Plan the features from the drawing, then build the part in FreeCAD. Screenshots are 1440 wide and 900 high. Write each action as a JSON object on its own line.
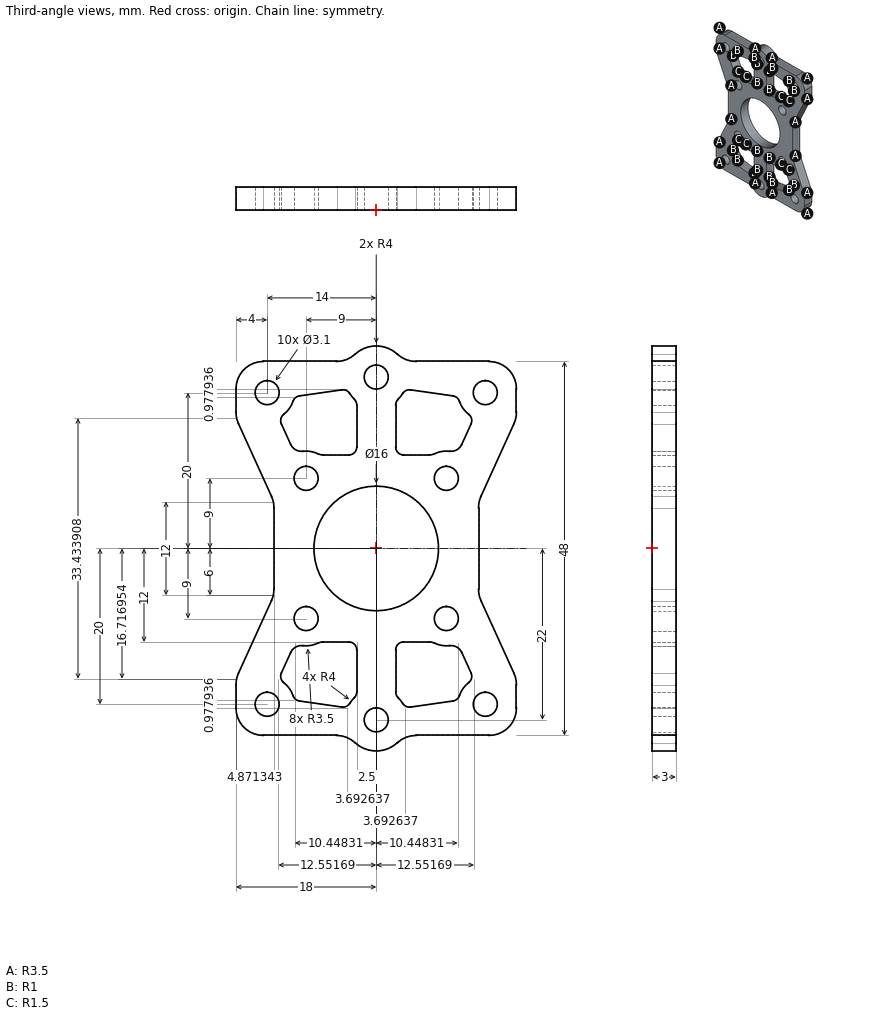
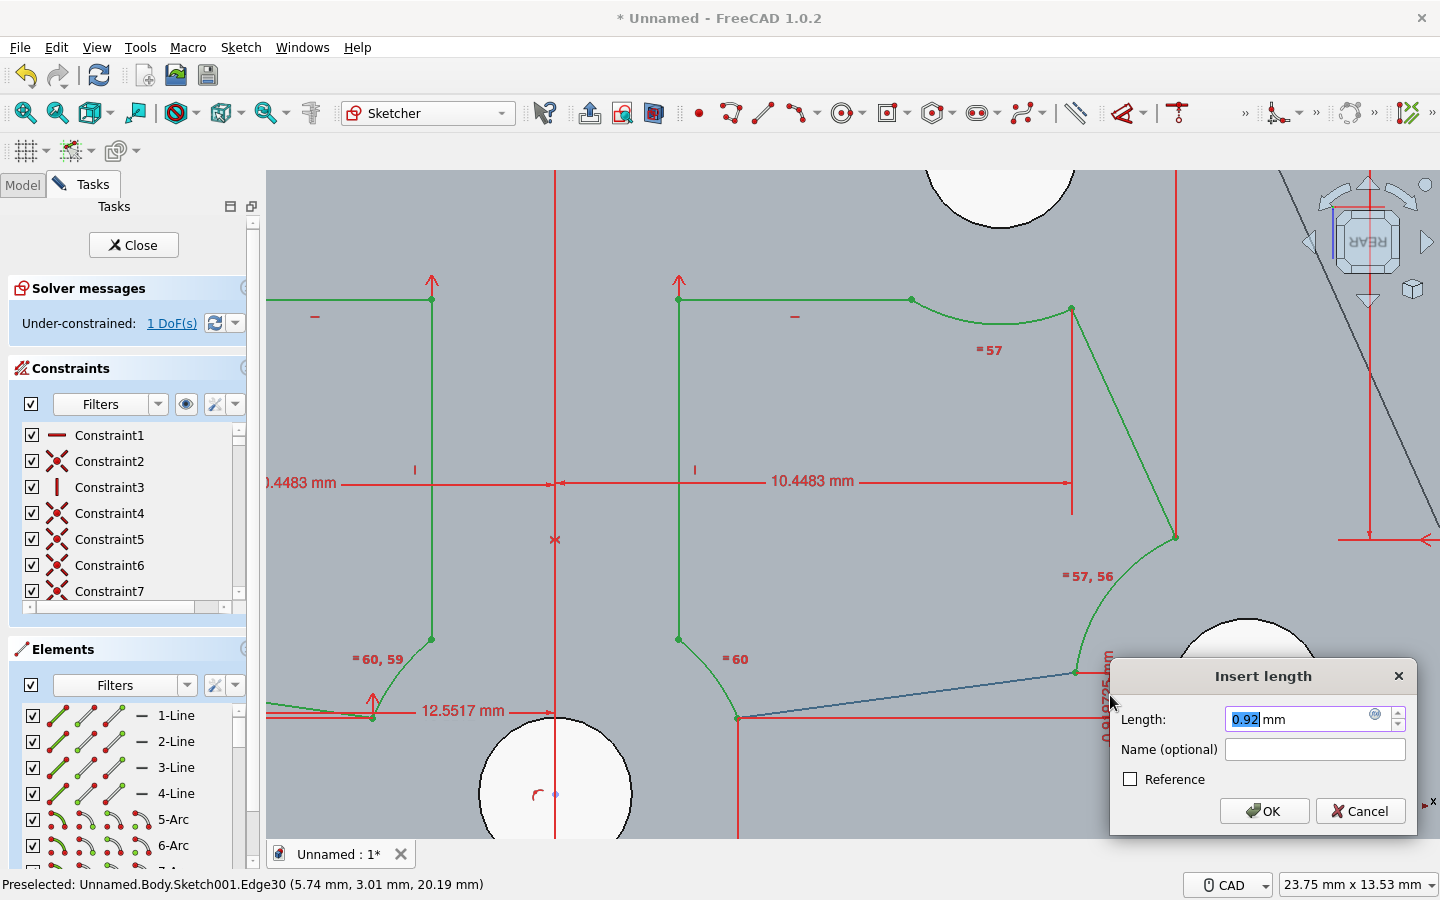
{"action": "type", "text": "0.977936"}
{"action": "key", "text": "Return"}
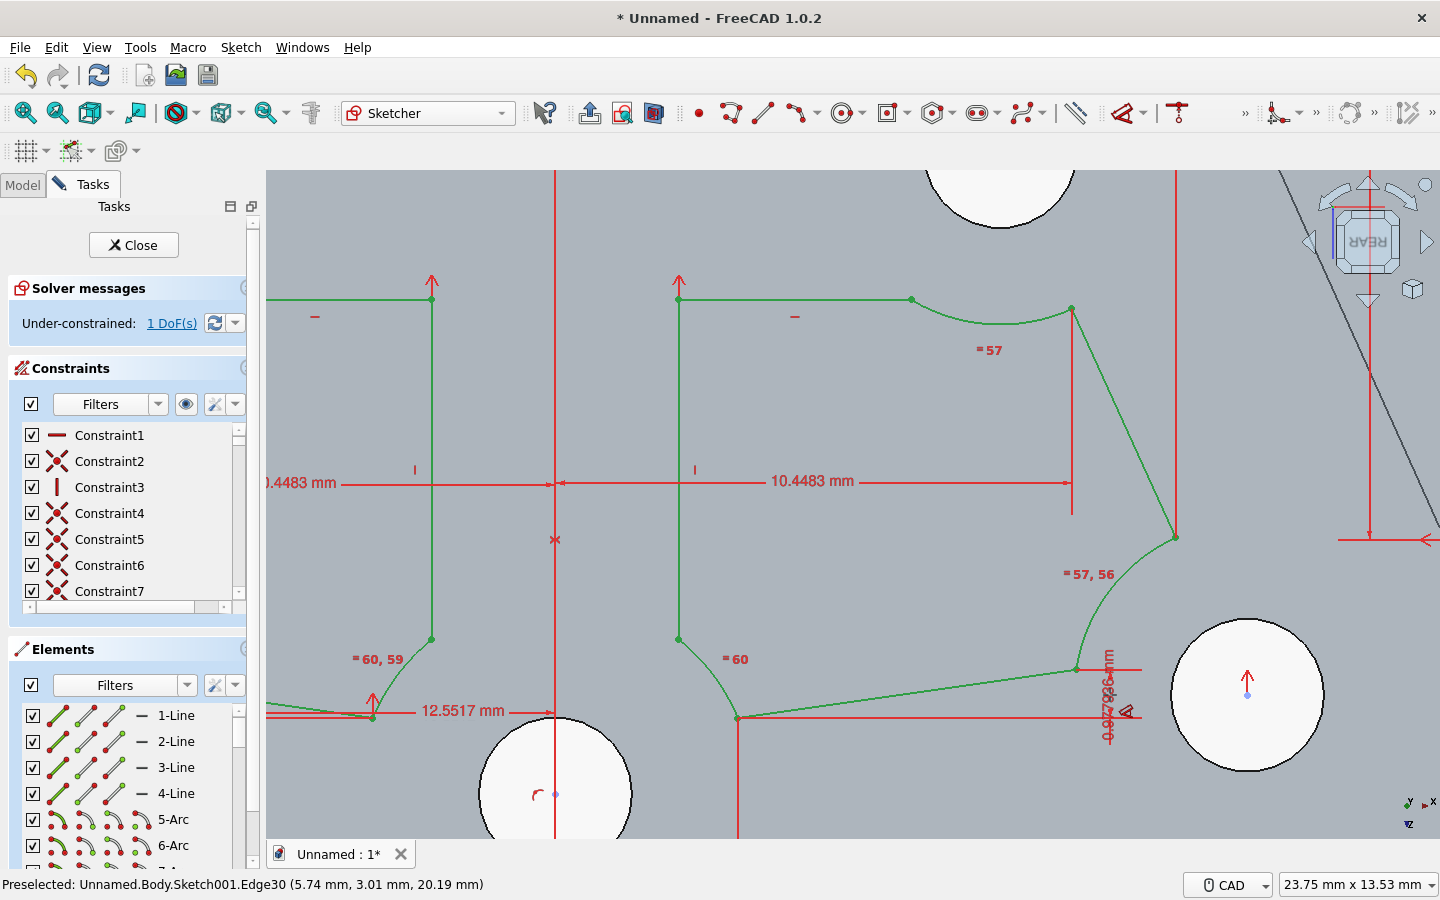
{"action": "scroll", "coordinate": [842, 706], "scroll_direction": "down", "scroll_amount": 8}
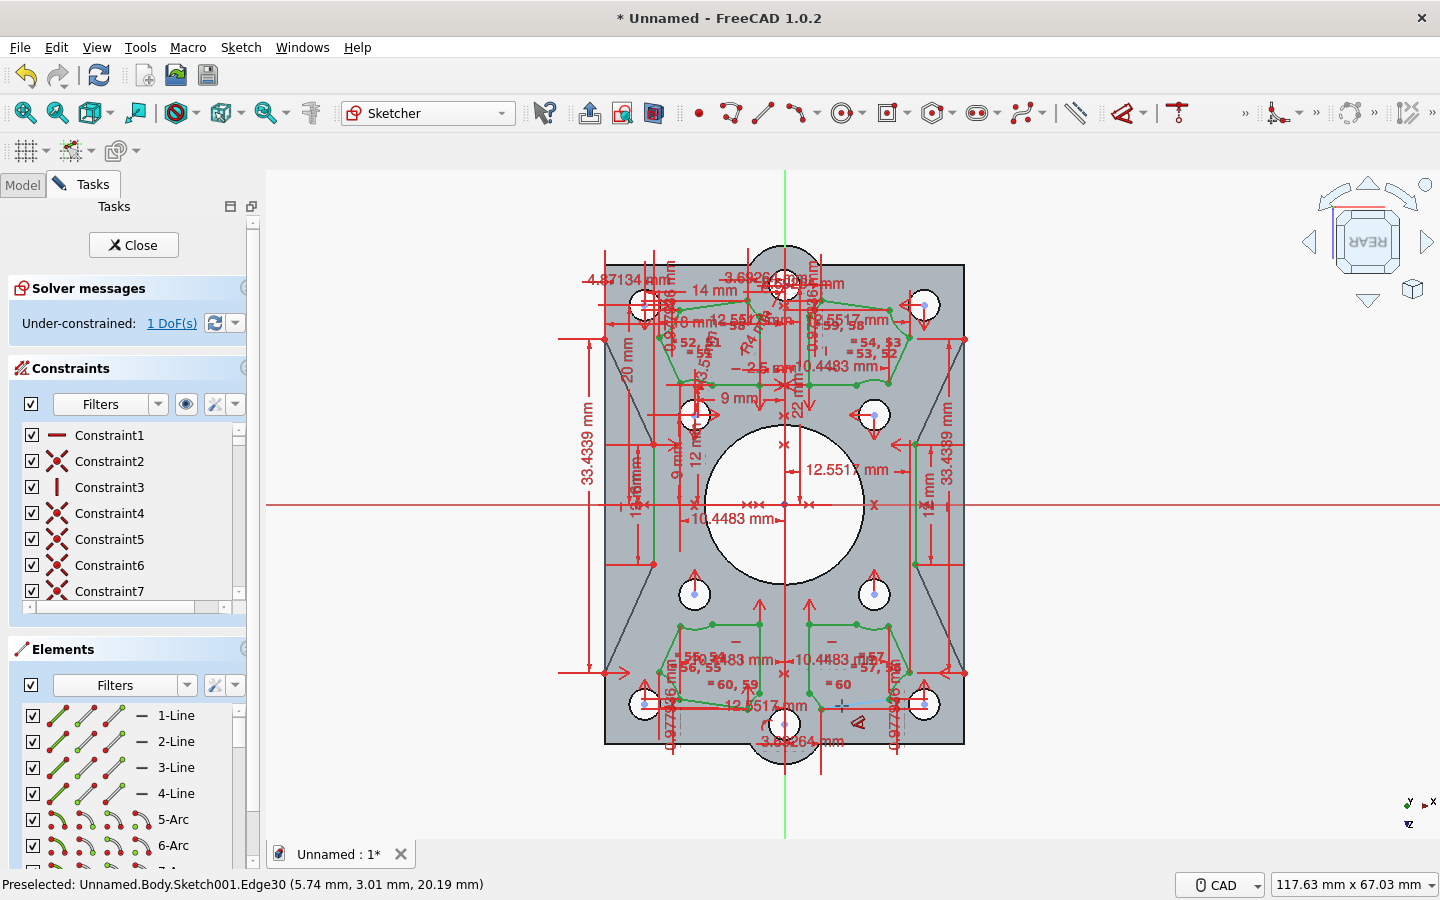
{"action": "left_click", "coordinate": [605, 339]}
{"action": "left_click", "coordinate": [571, 422]}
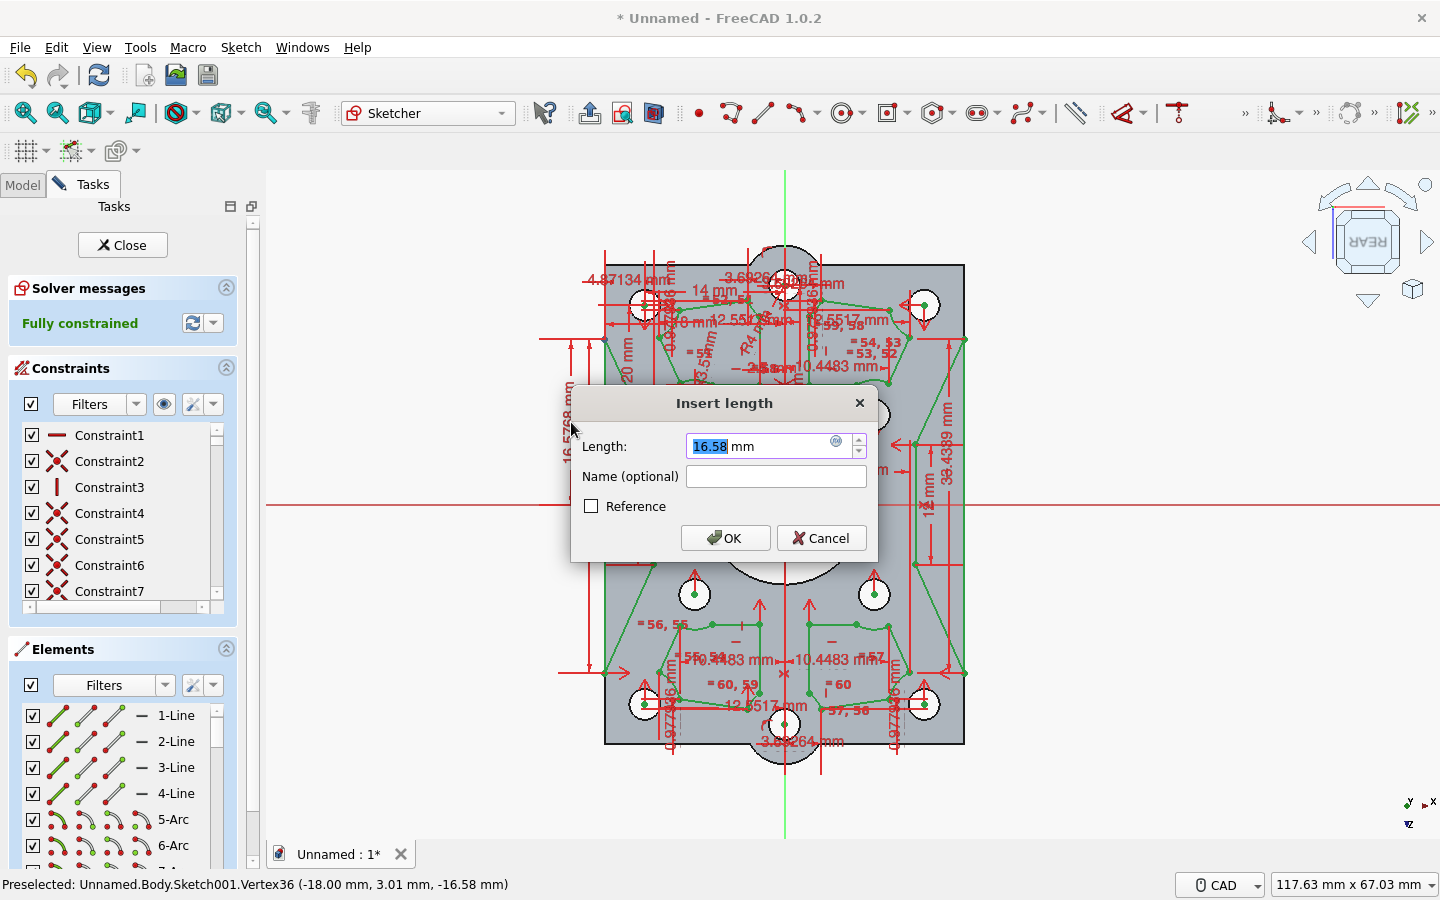
{"action": "type", "text": "16.716954"}
{"action": "key", "text": "Return"}
{"action": "key", "text": "Escape"}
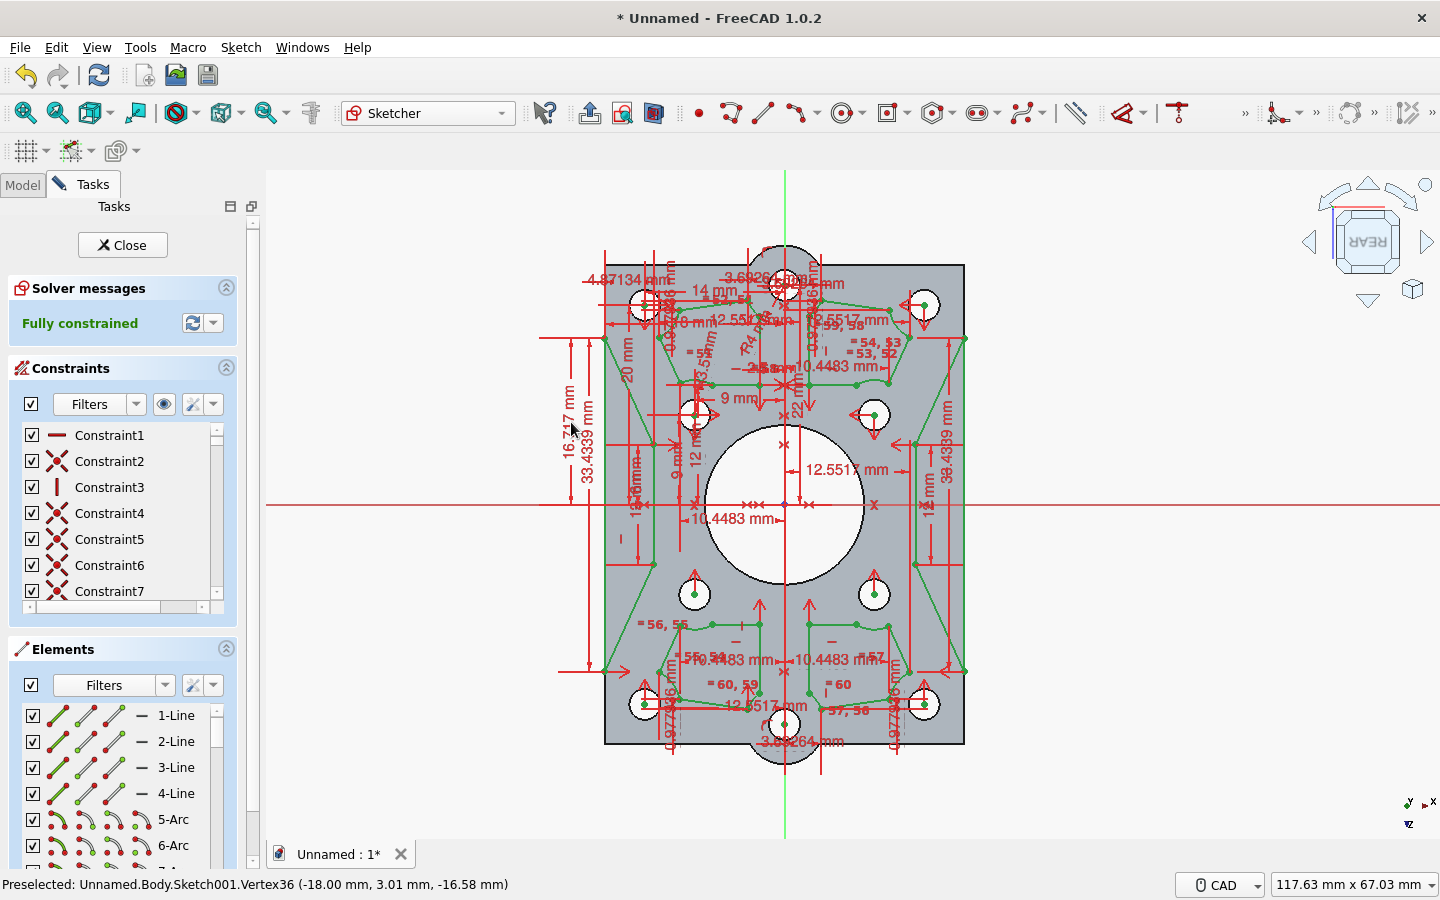
{"action": "left_click", "coordinate": [123, 245]}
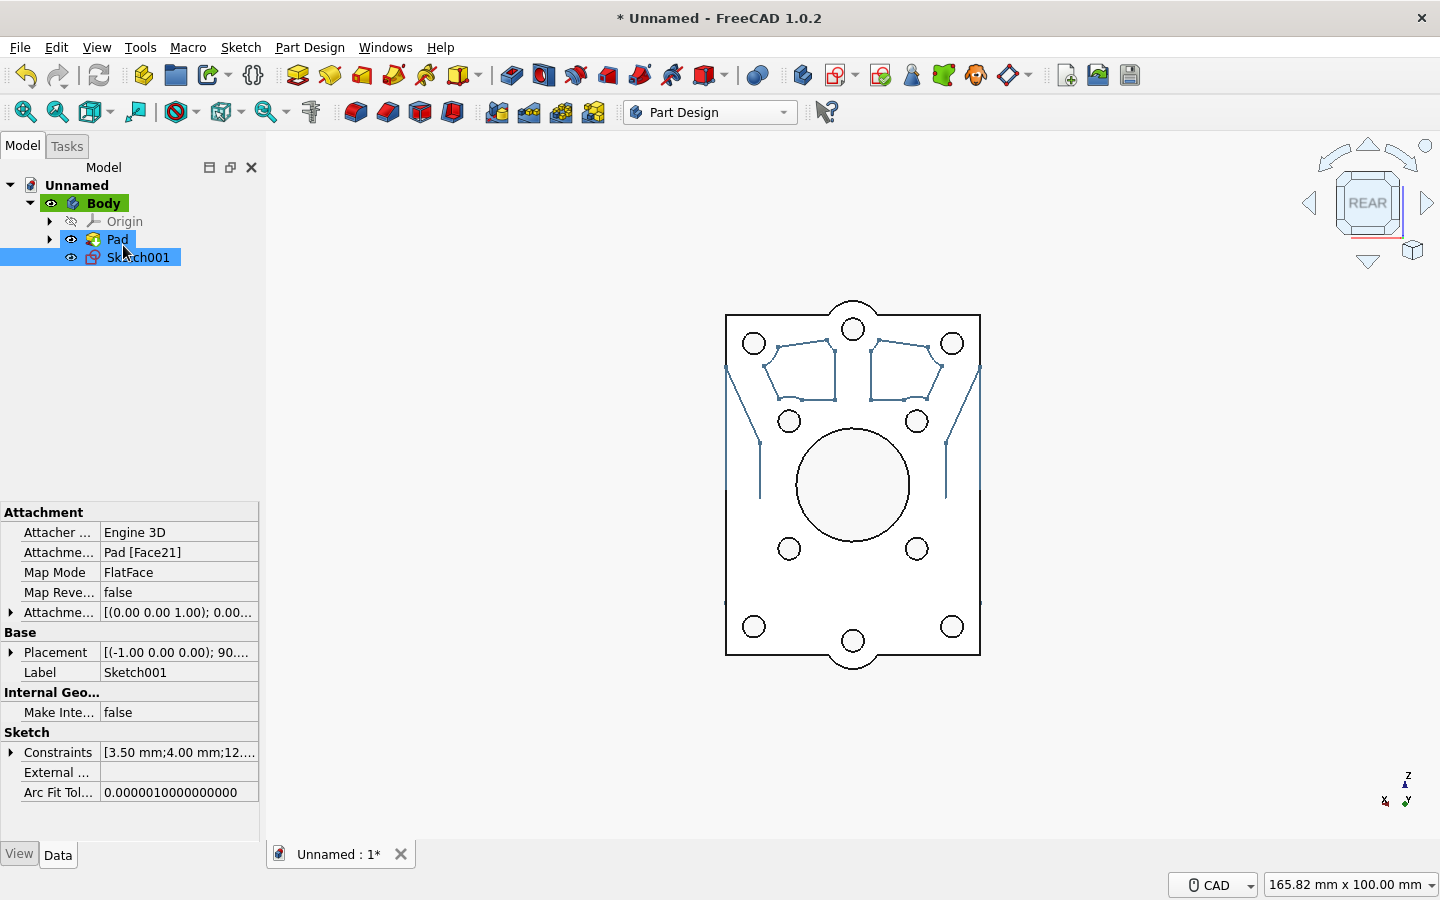
{"action": "left_click", "coordinate": [512, 76]}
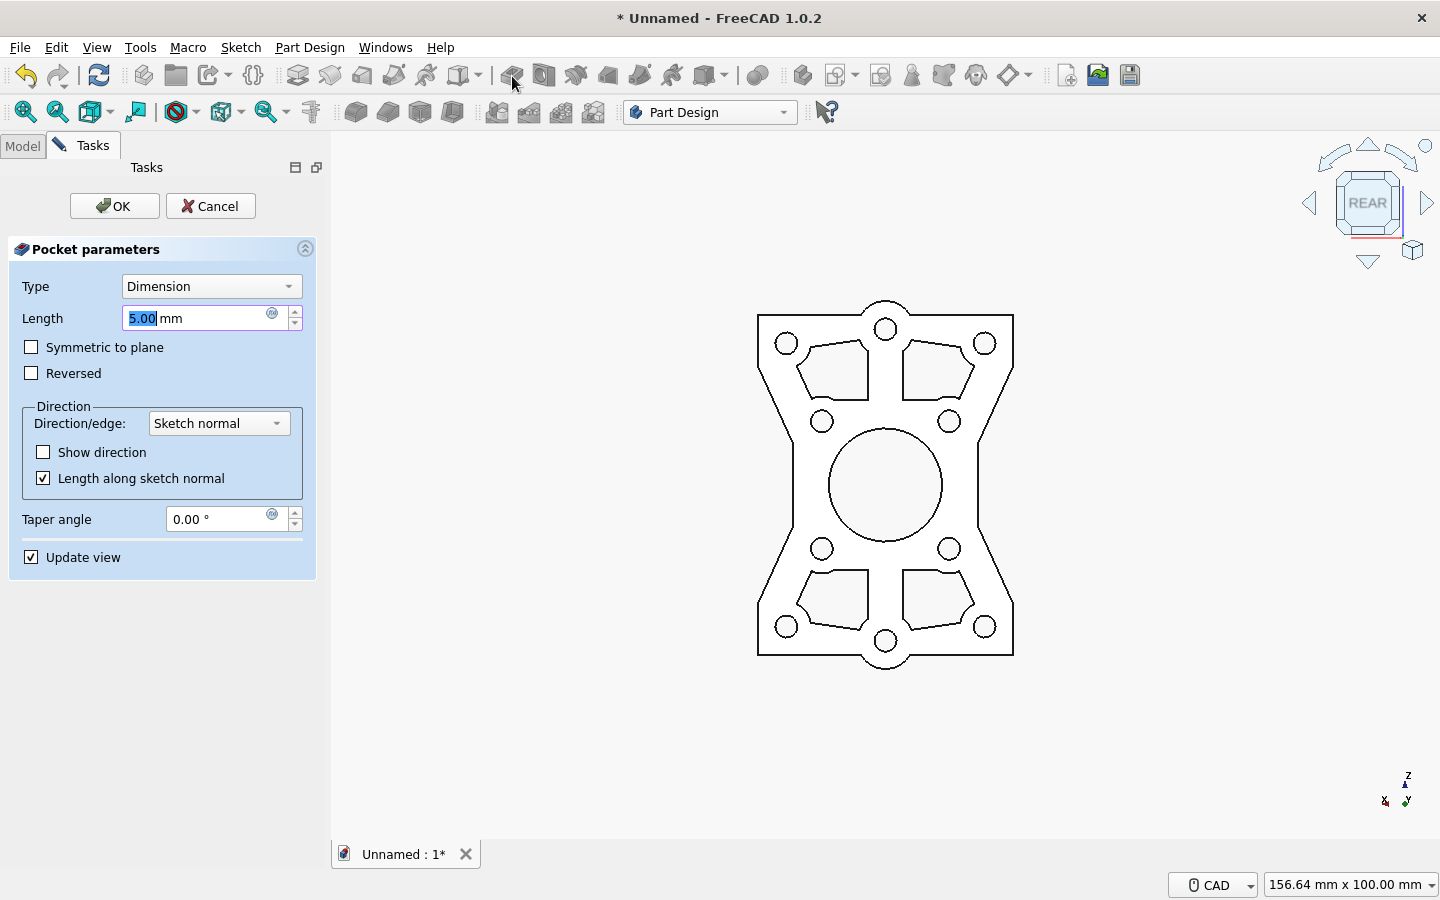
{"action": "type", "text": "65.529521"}
{"action": "key", "text": "Tab"}